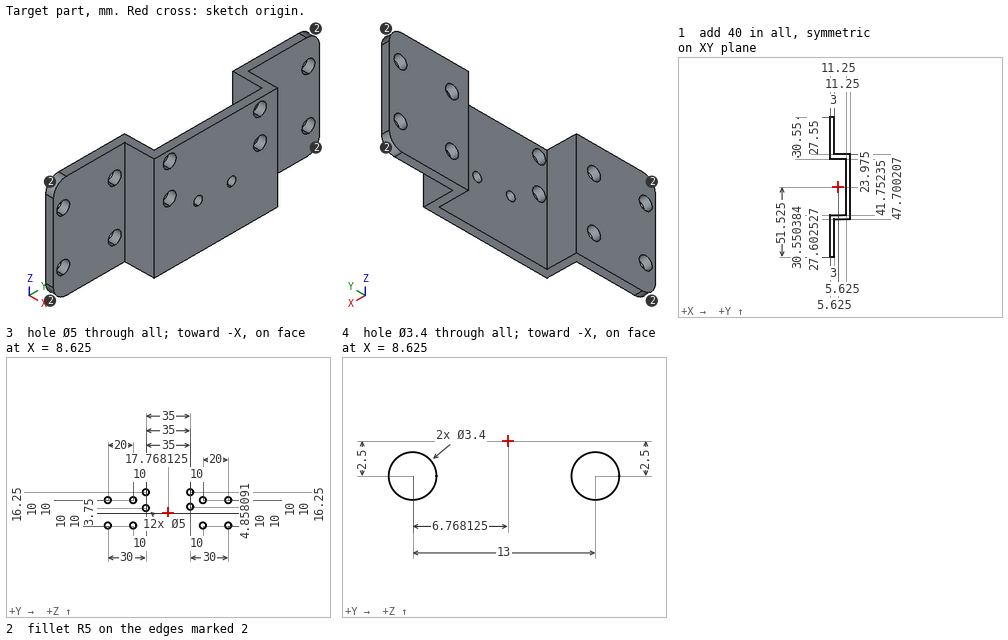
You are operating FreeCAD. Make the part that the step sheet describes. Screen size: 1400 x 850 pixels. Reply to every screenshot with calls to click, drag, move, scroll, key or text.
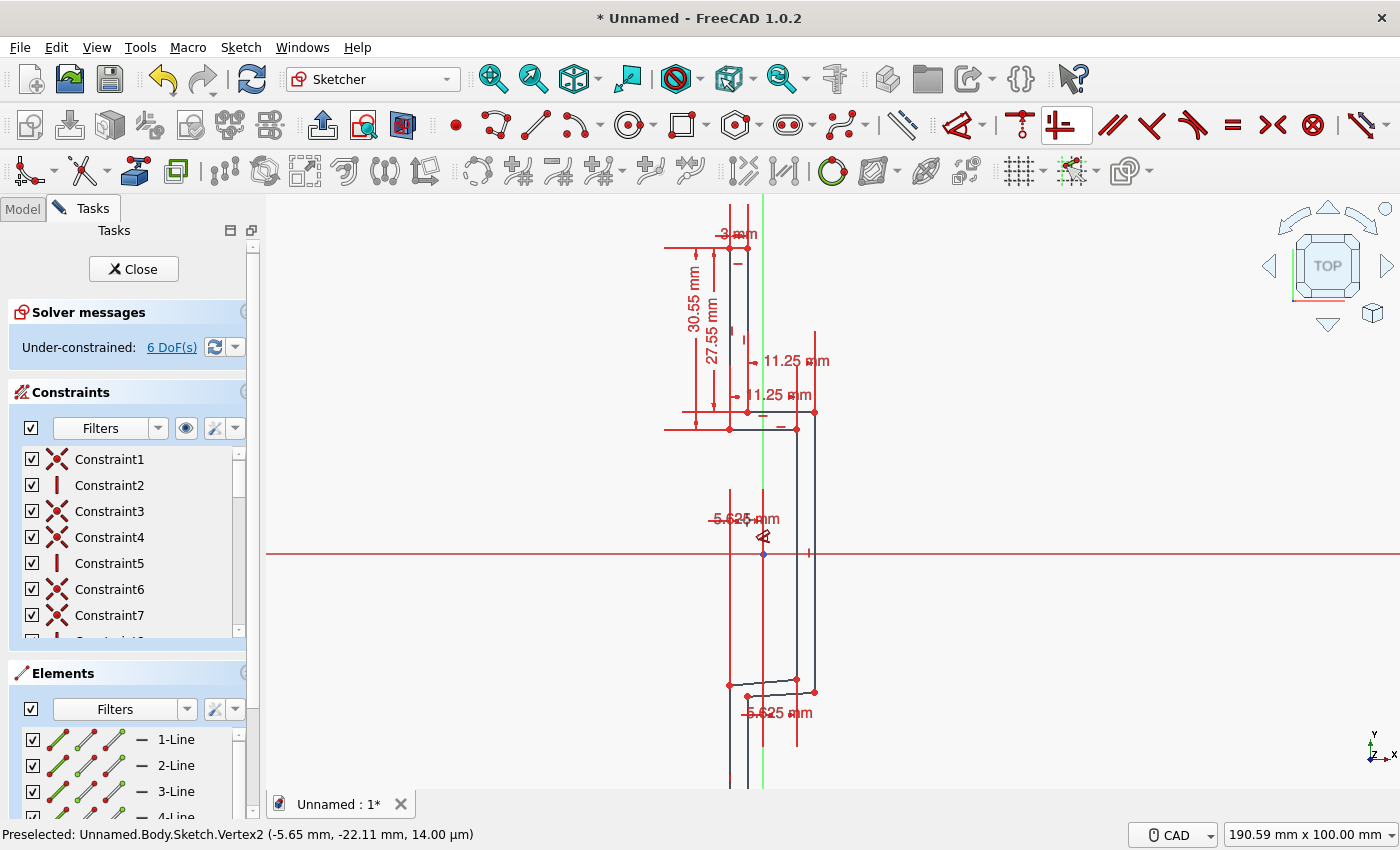
scroll(749, 364, down, 2)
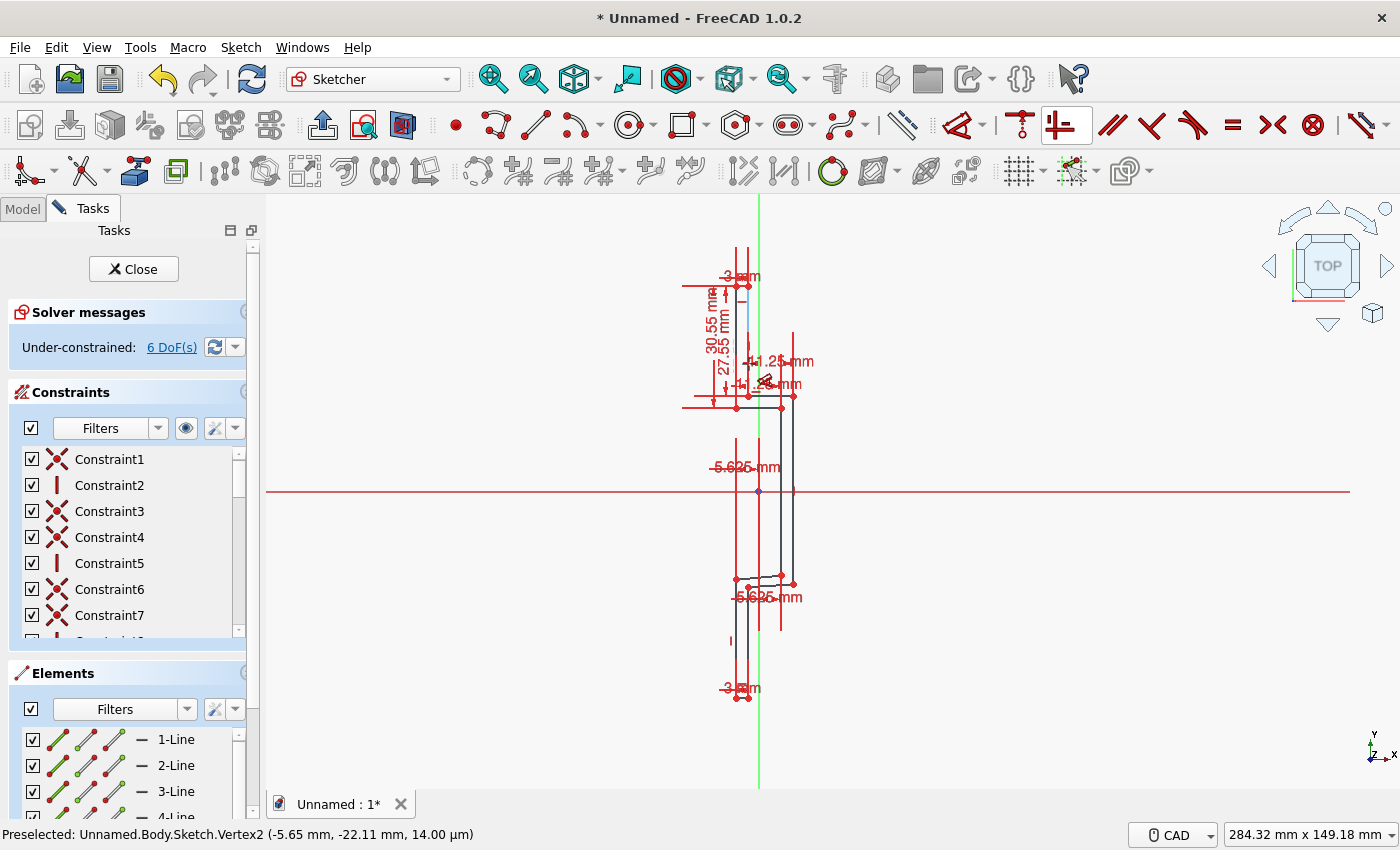
click(736, 698)
click(702, 547)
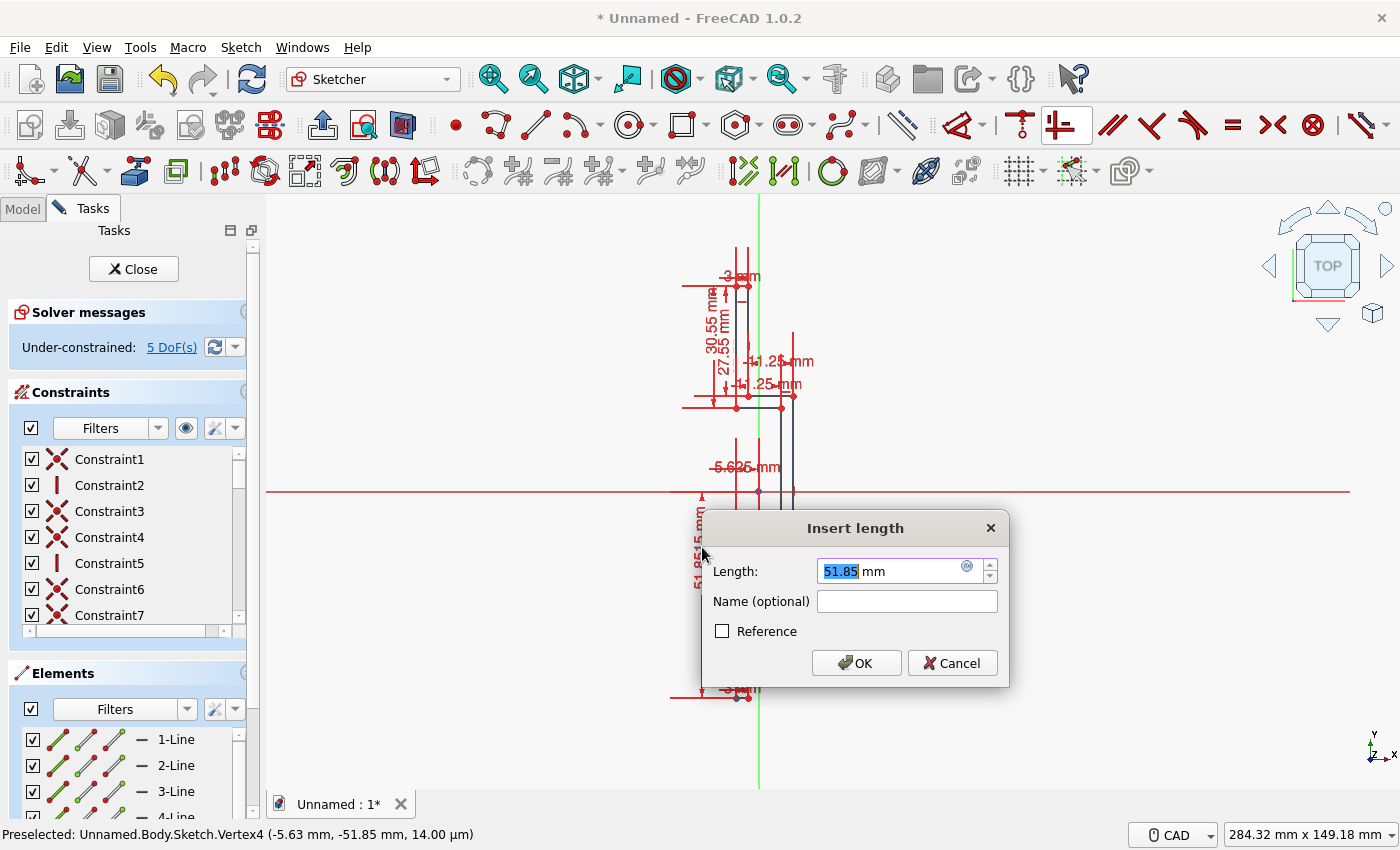
text(51.525)
key(Return)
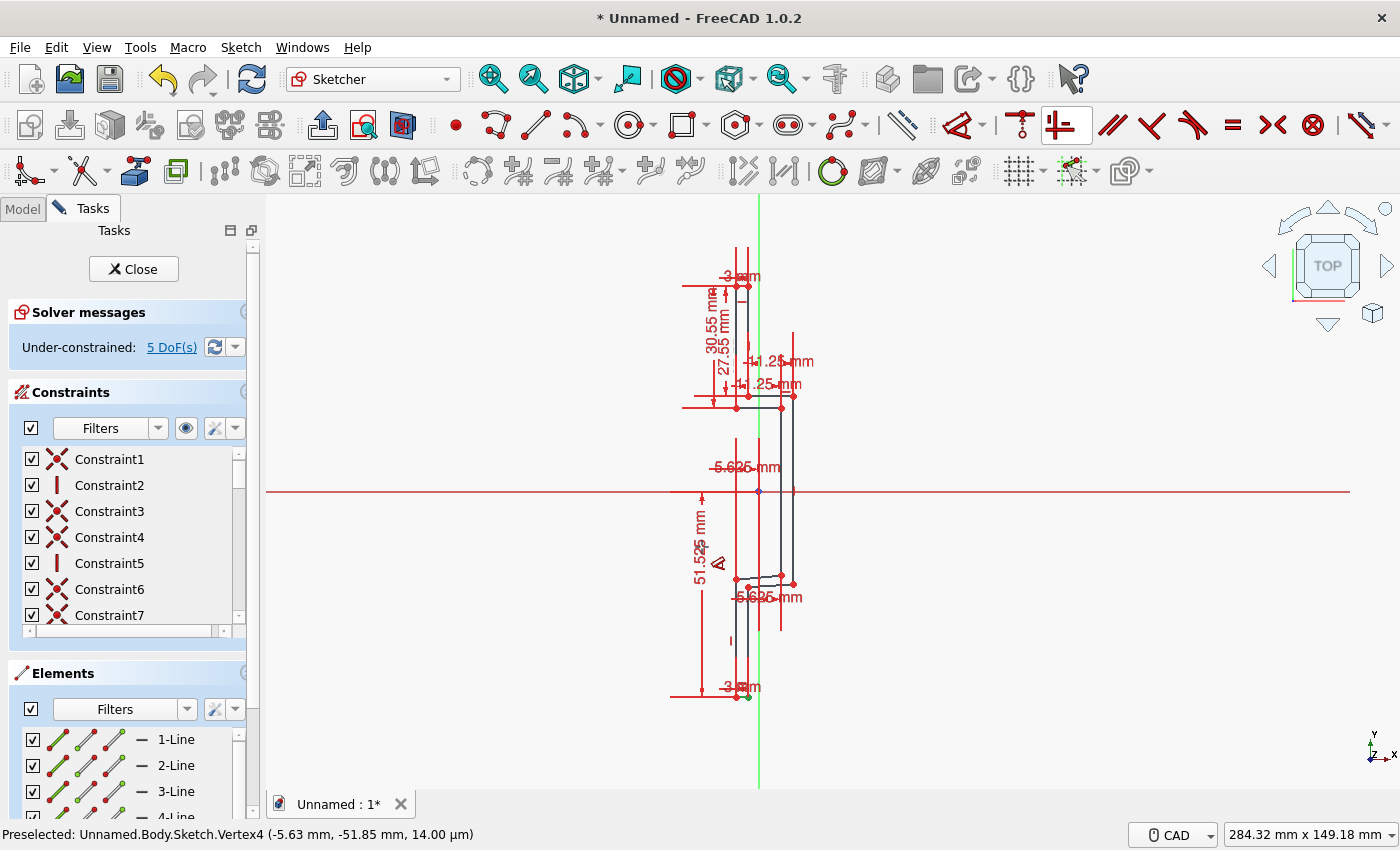
click(793, 396)
click(827, 444)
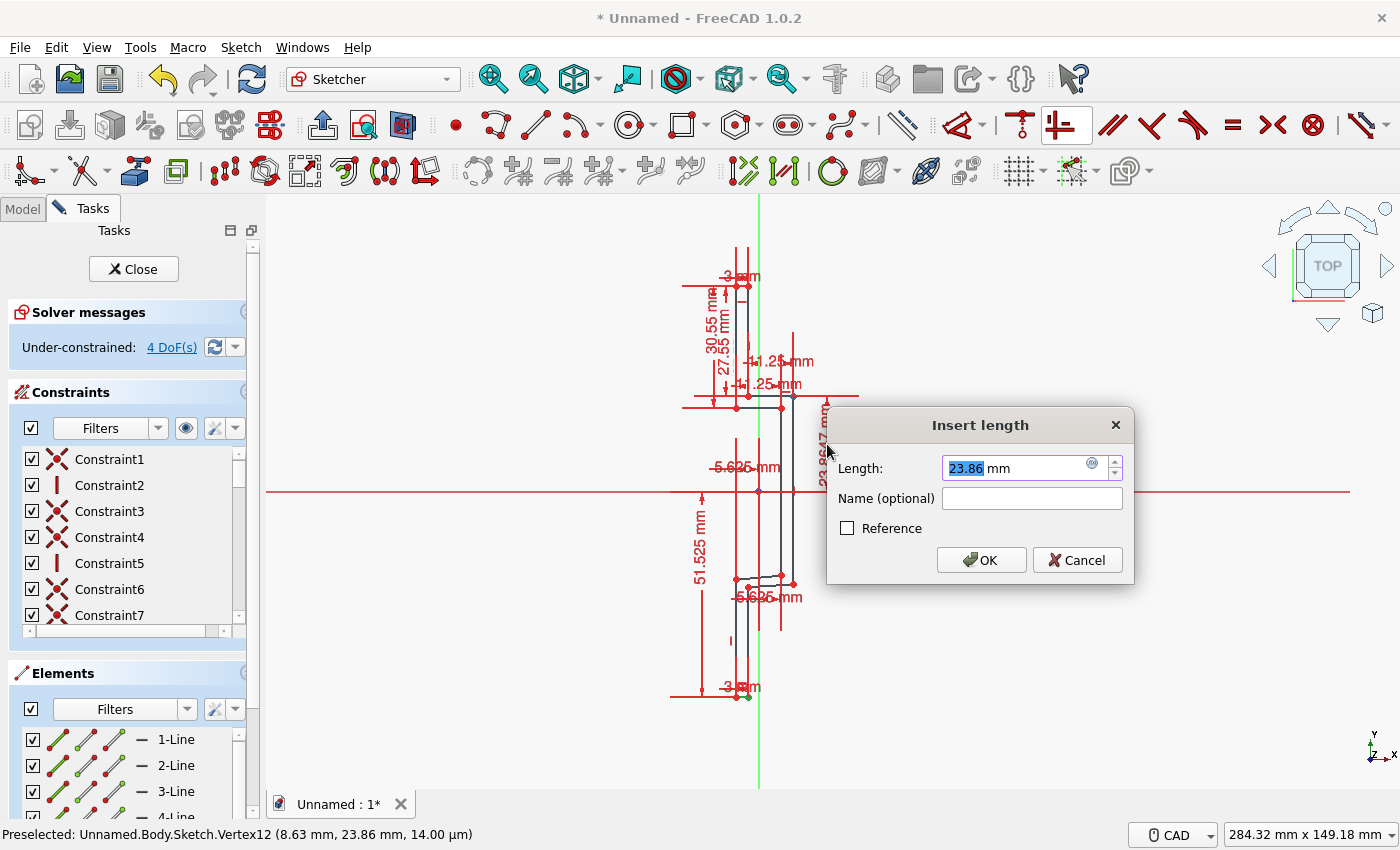
text(23.975)
key(Return)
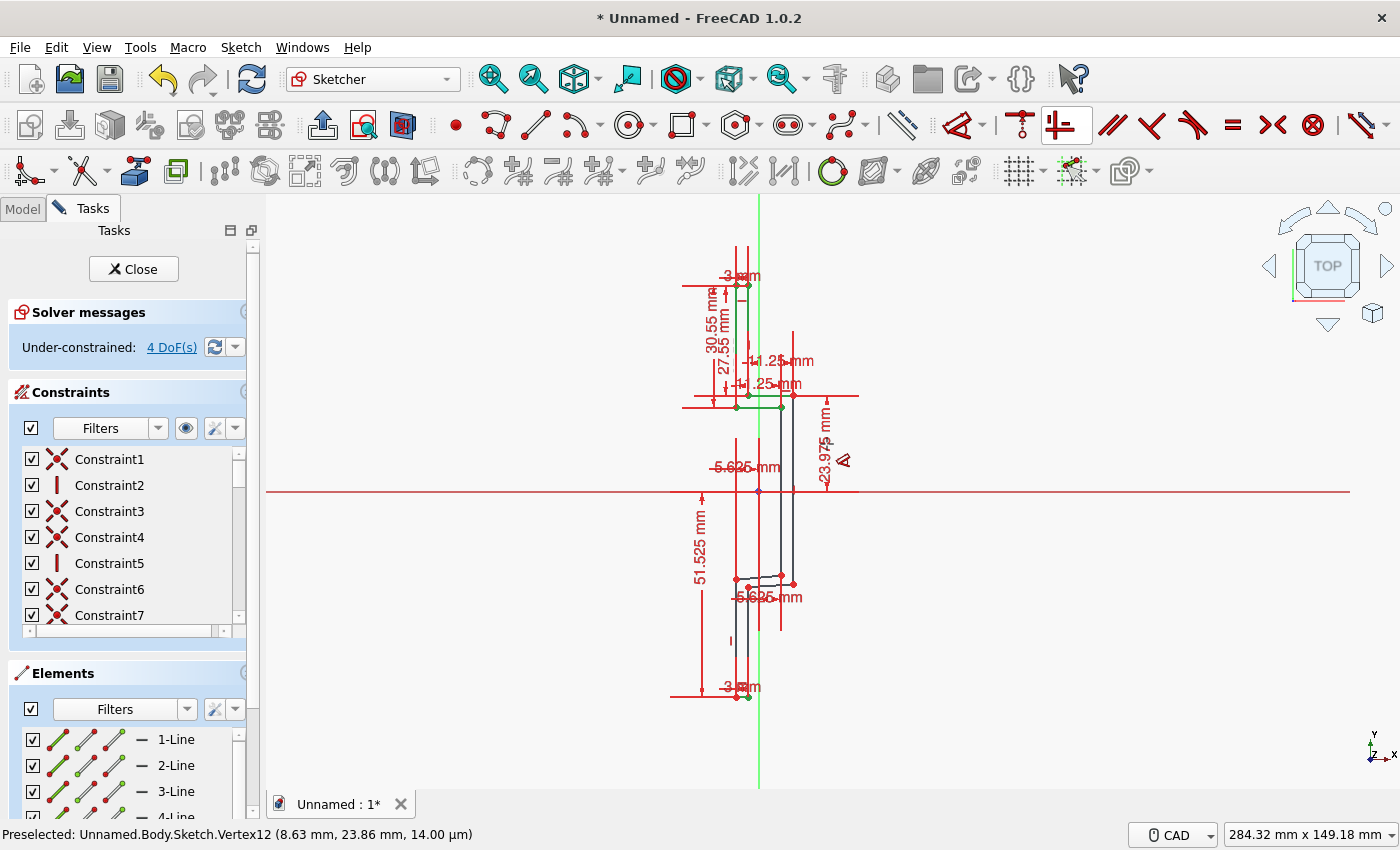
click(781, 458)
click(815, 530)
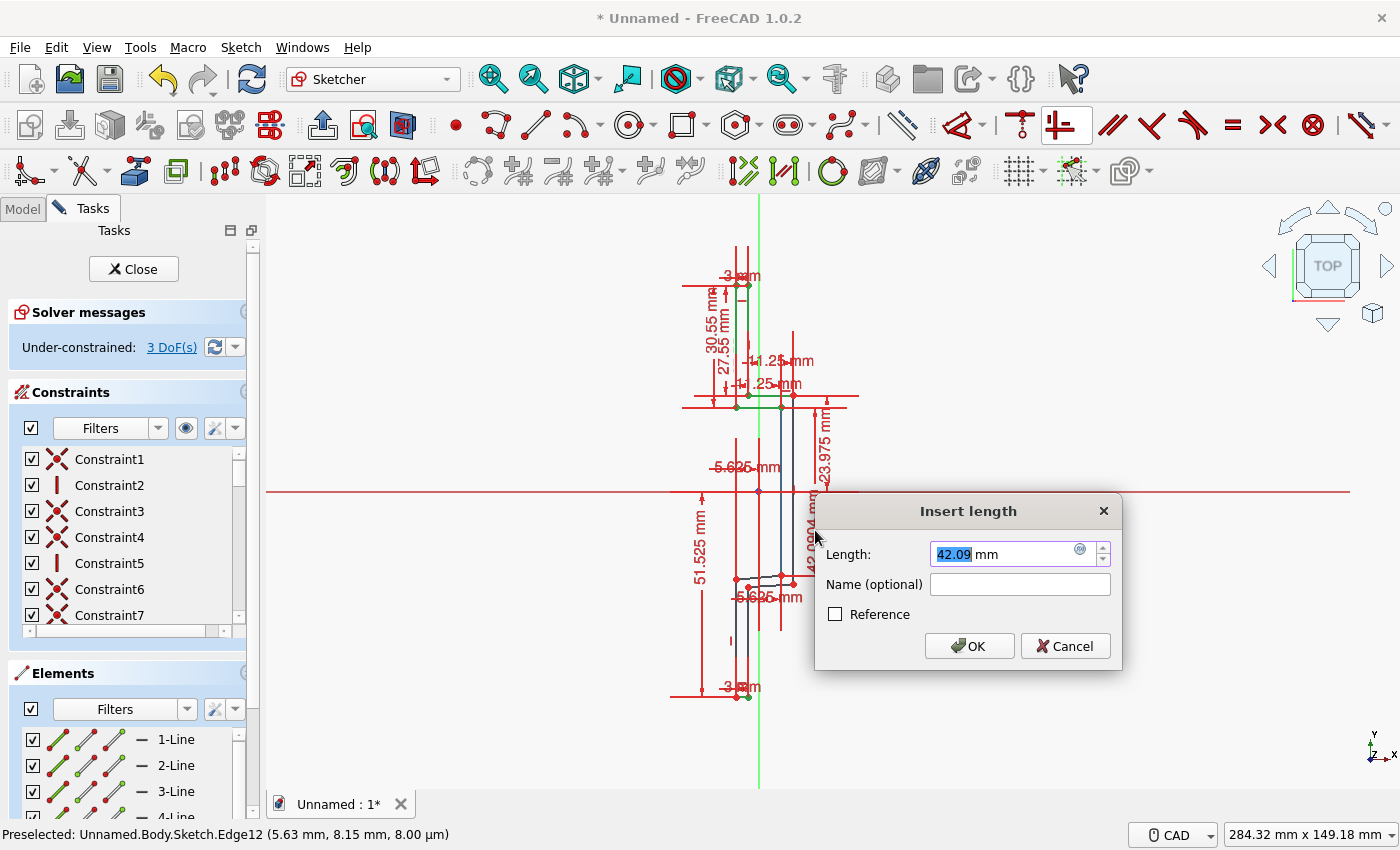
text(41.75235)
key(Return)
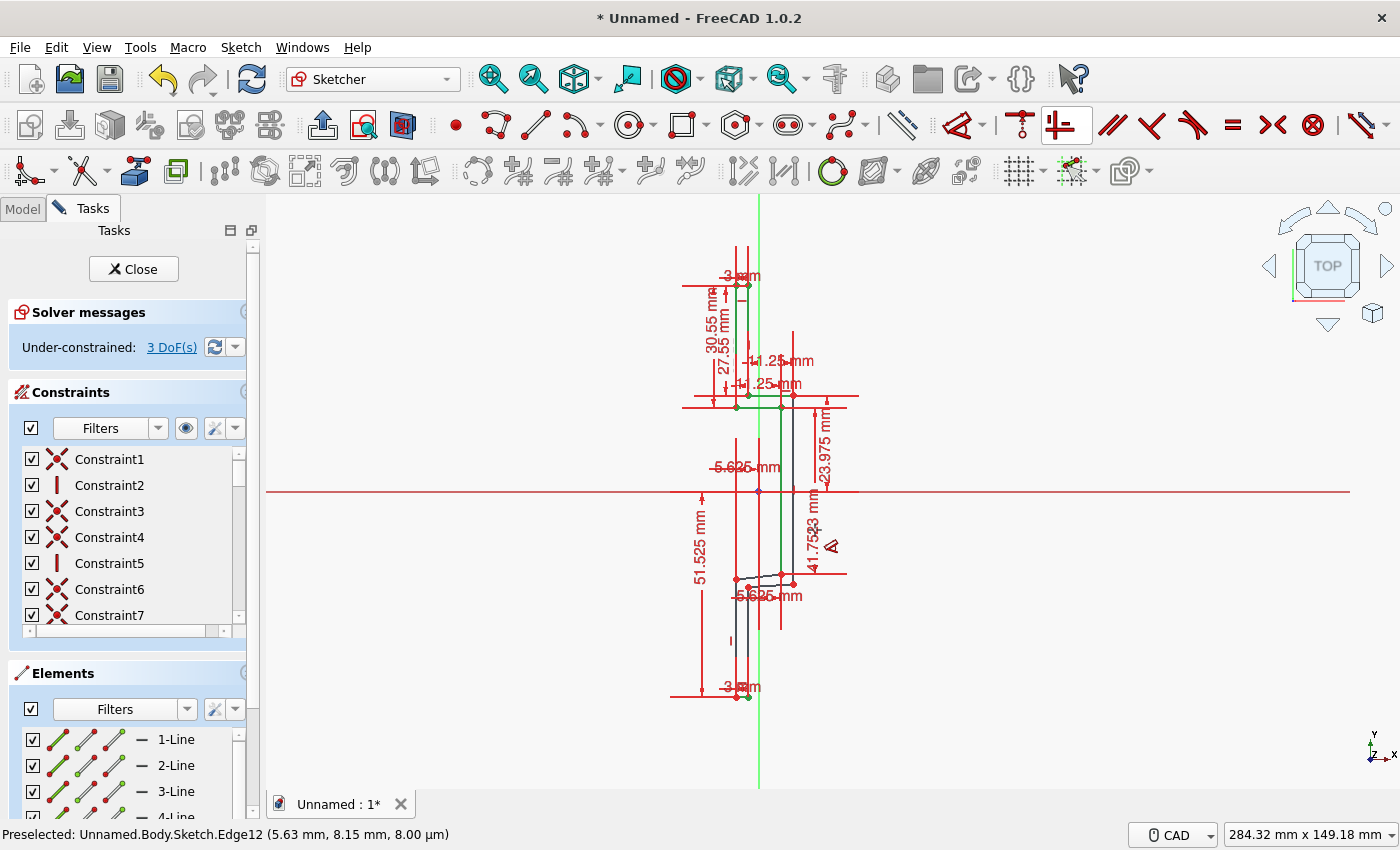
click(736, 615)
click(702, 638)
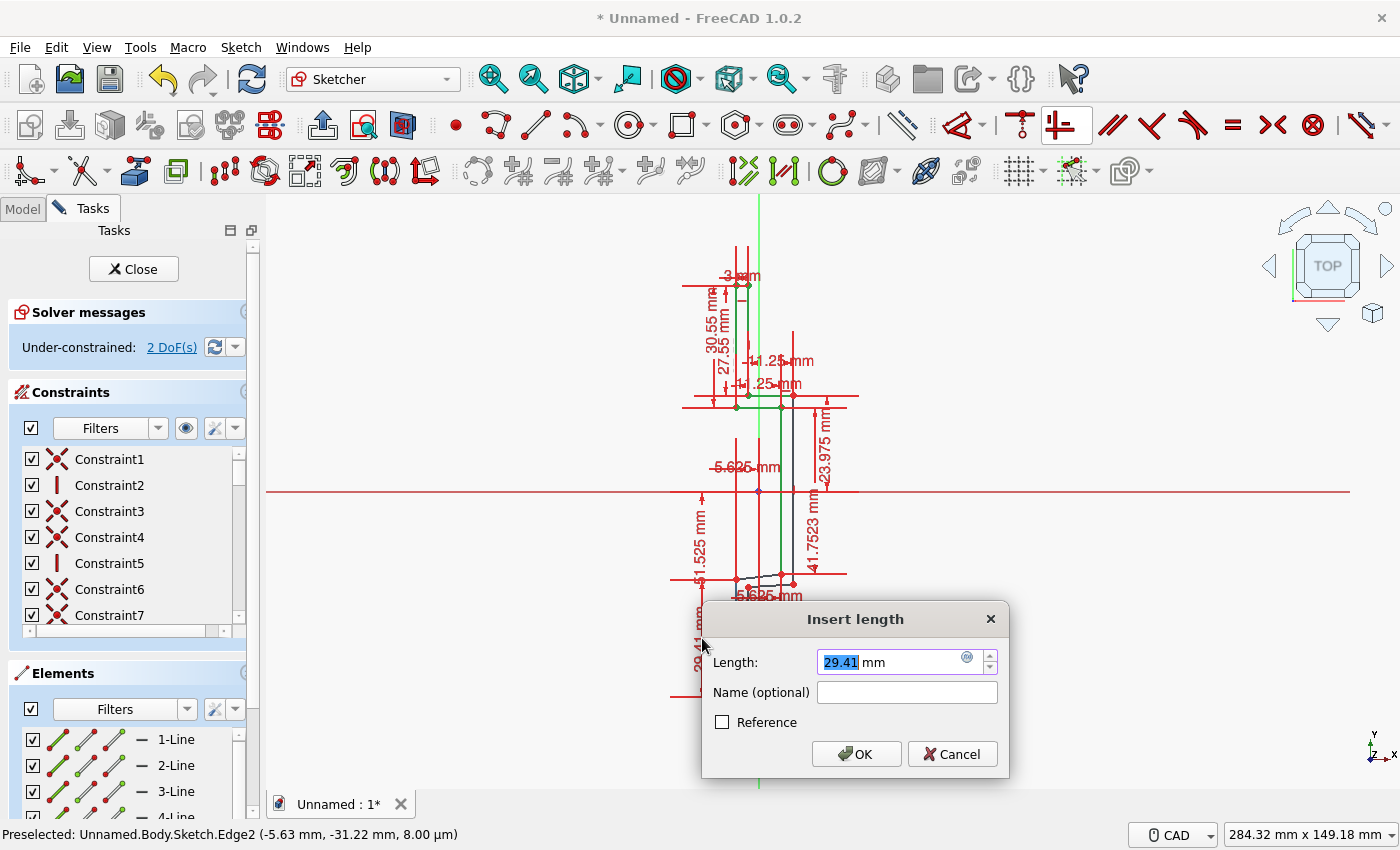
text(30.550384)
key(Return)